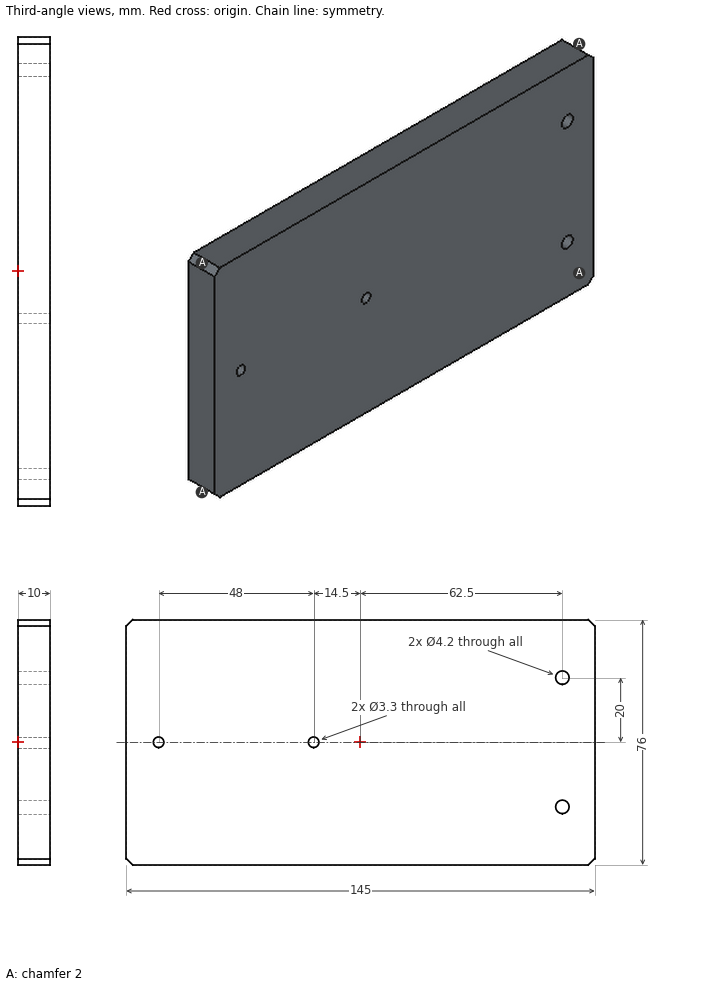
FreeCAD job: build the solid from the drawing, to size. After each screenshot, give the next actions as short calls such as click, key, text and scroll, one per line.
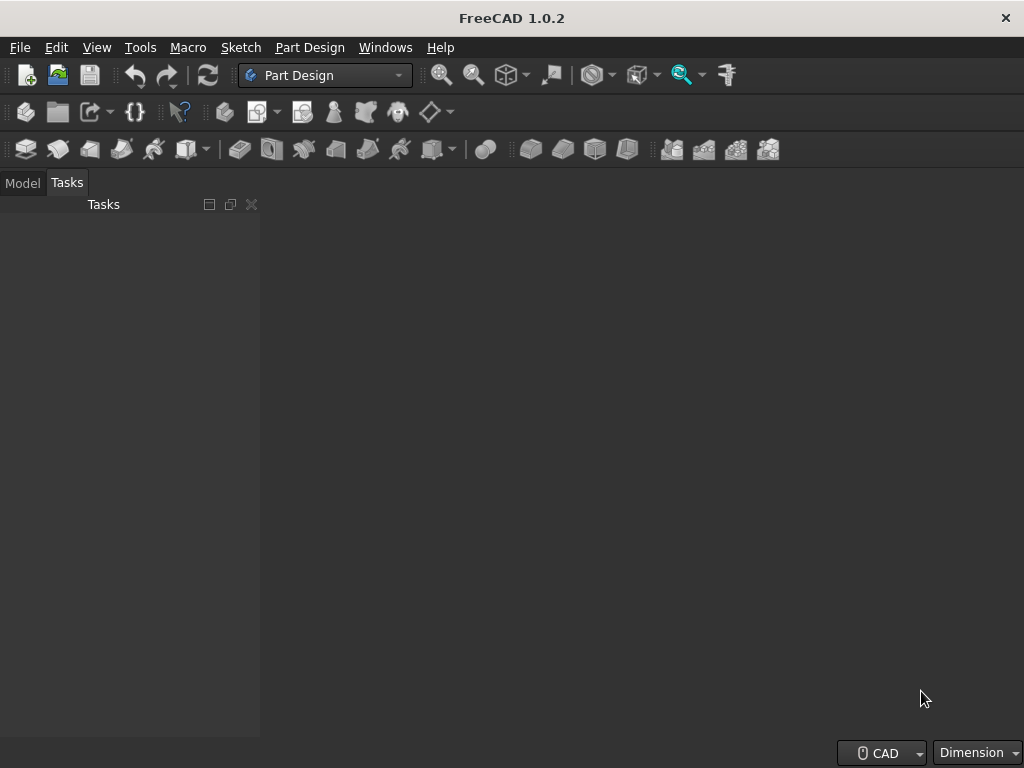
key(ctrl+n)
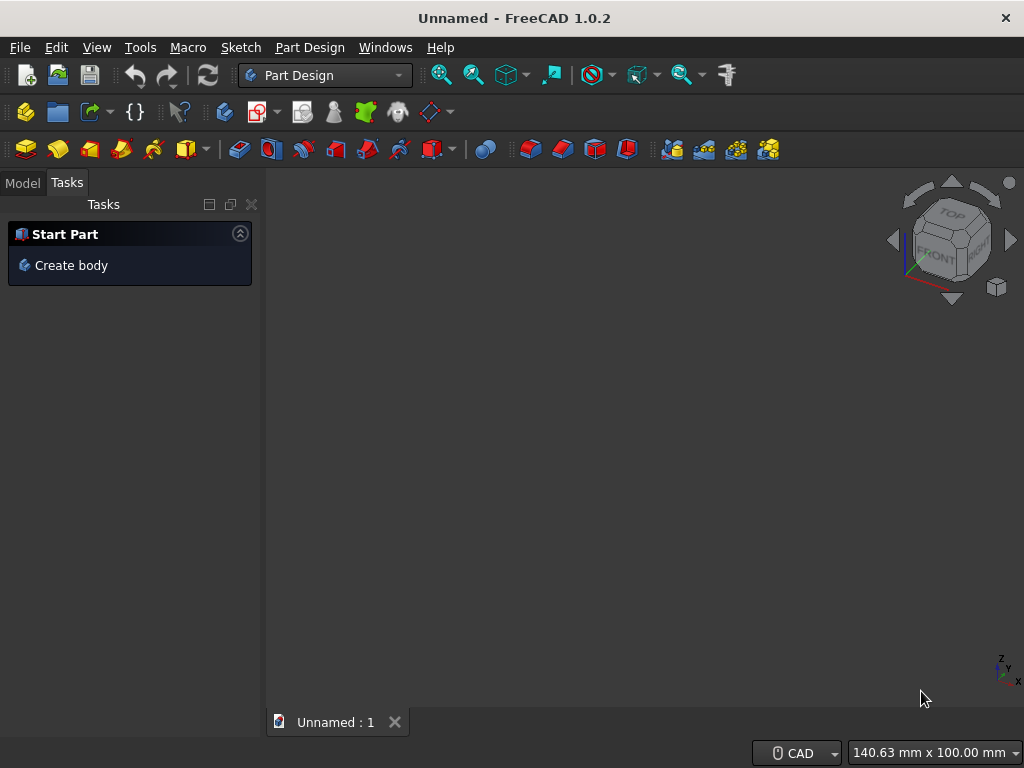
click(258, 112)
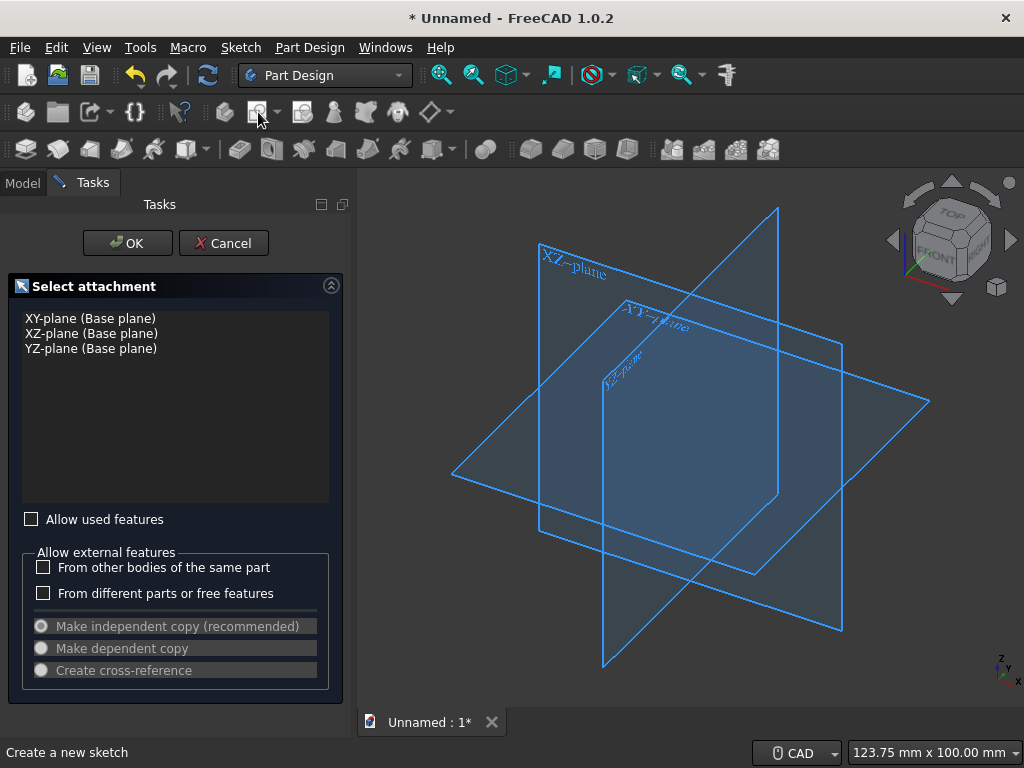
click(82, 348)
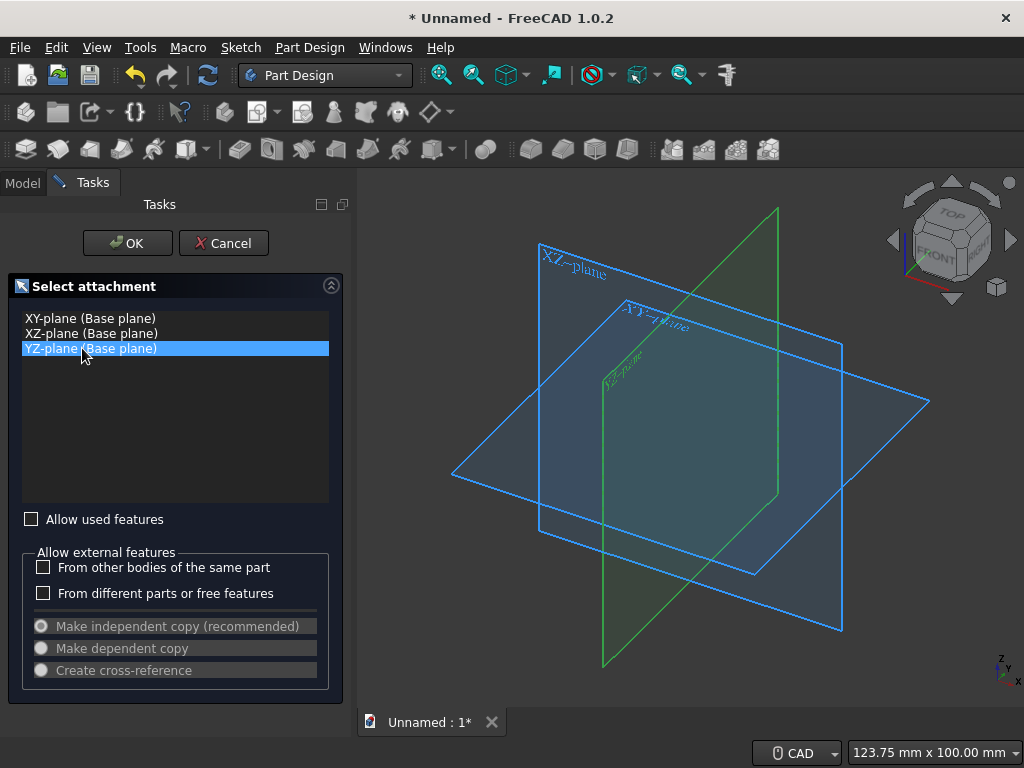
click(128, 243)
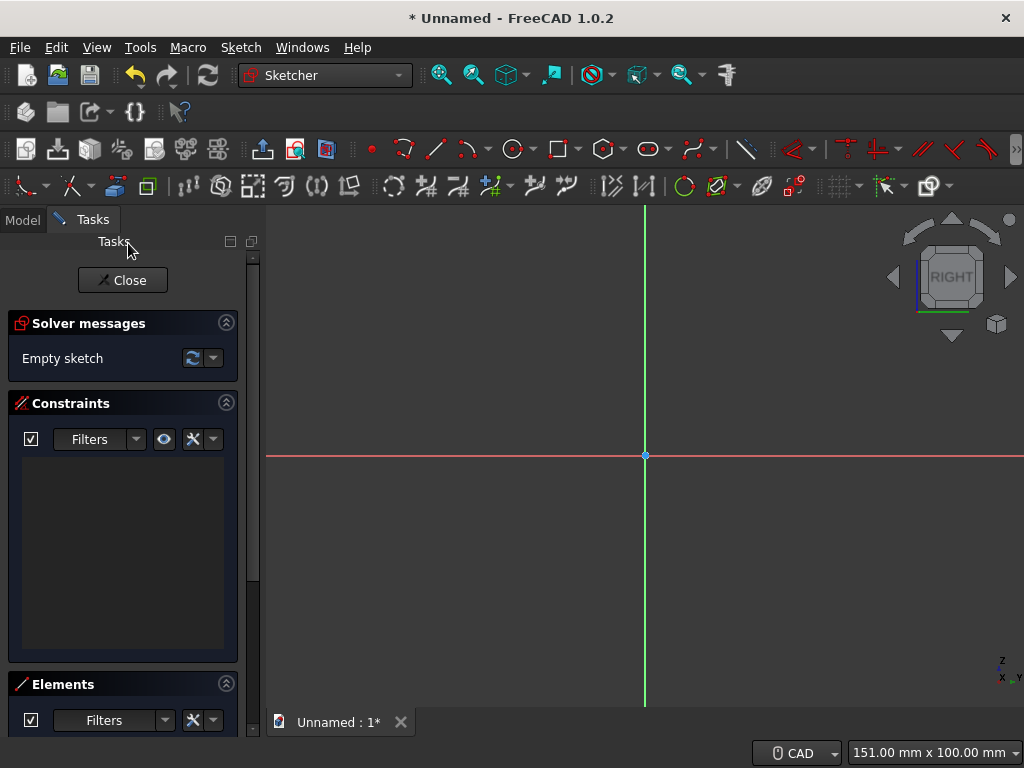
scroll(493, 456, down, 3)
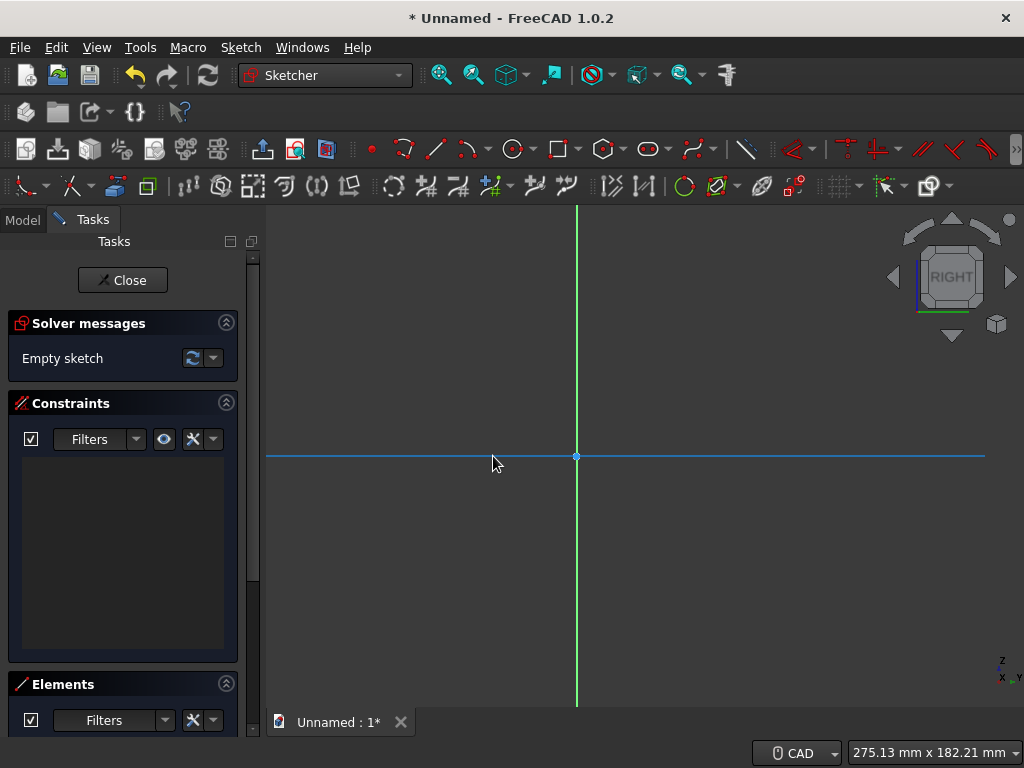
key(g)
key(v)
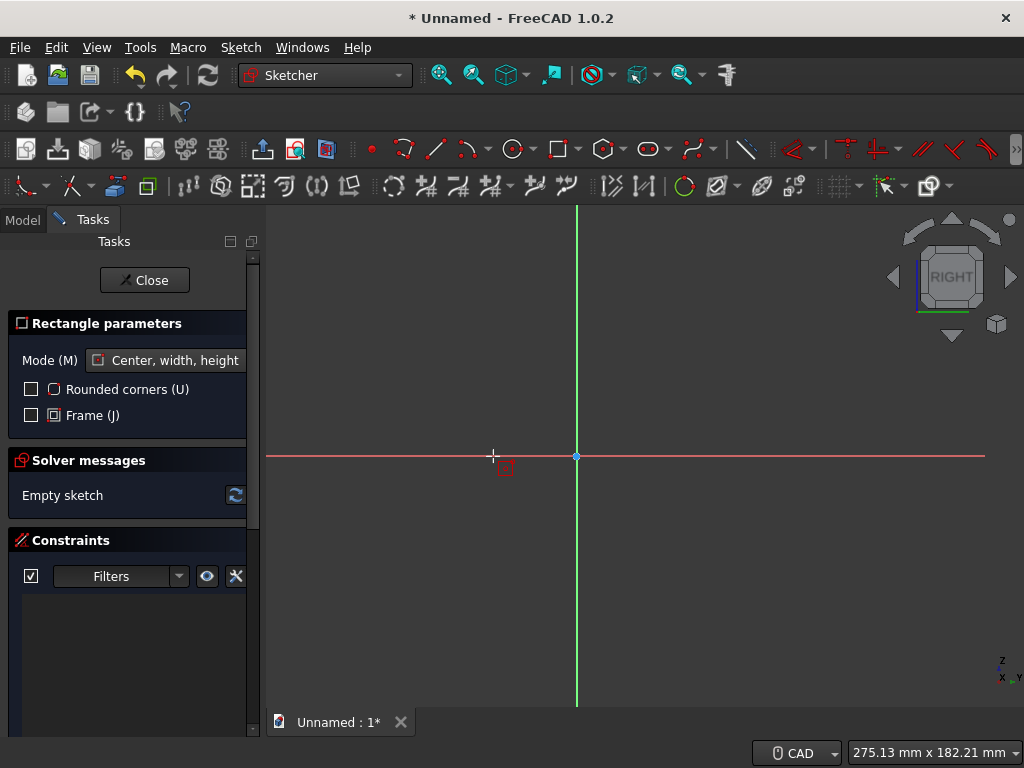
click(577, 456)
click(776, 352)
key(Escape)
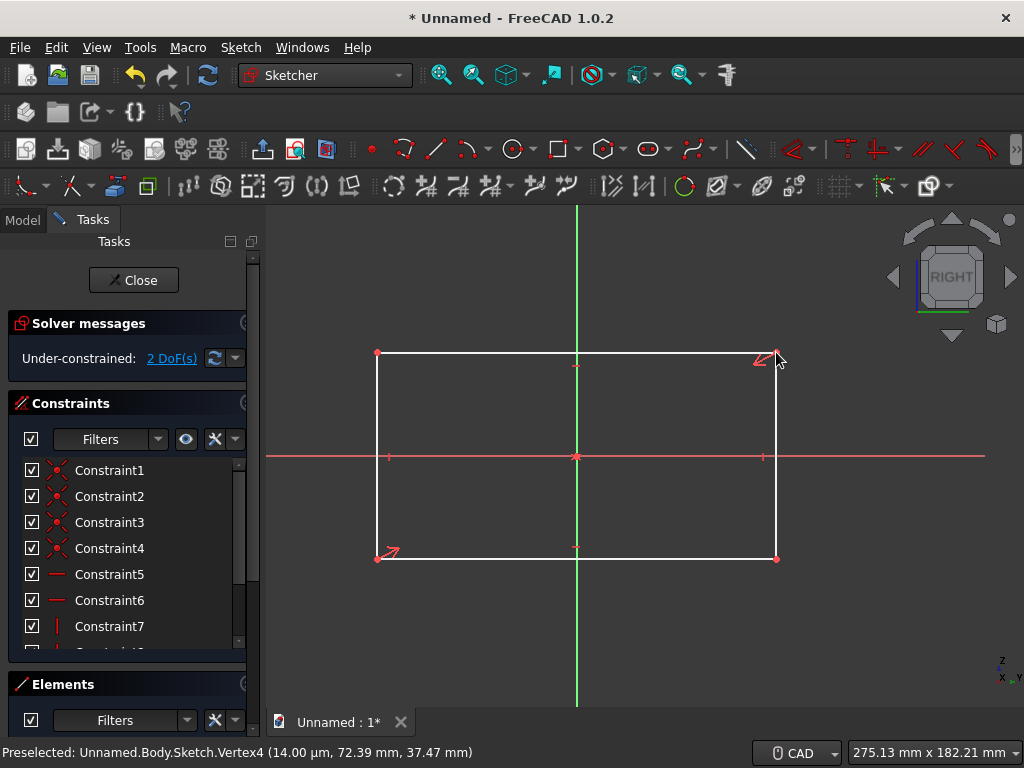
key(d)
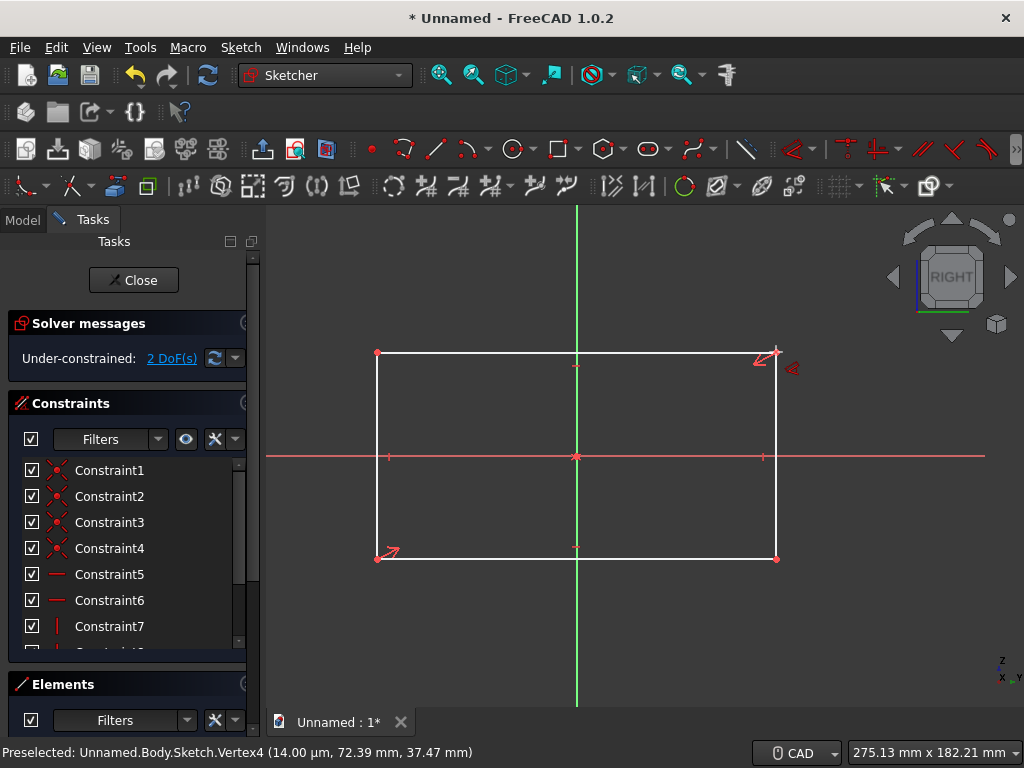
click(776, 498)
click(810, 409)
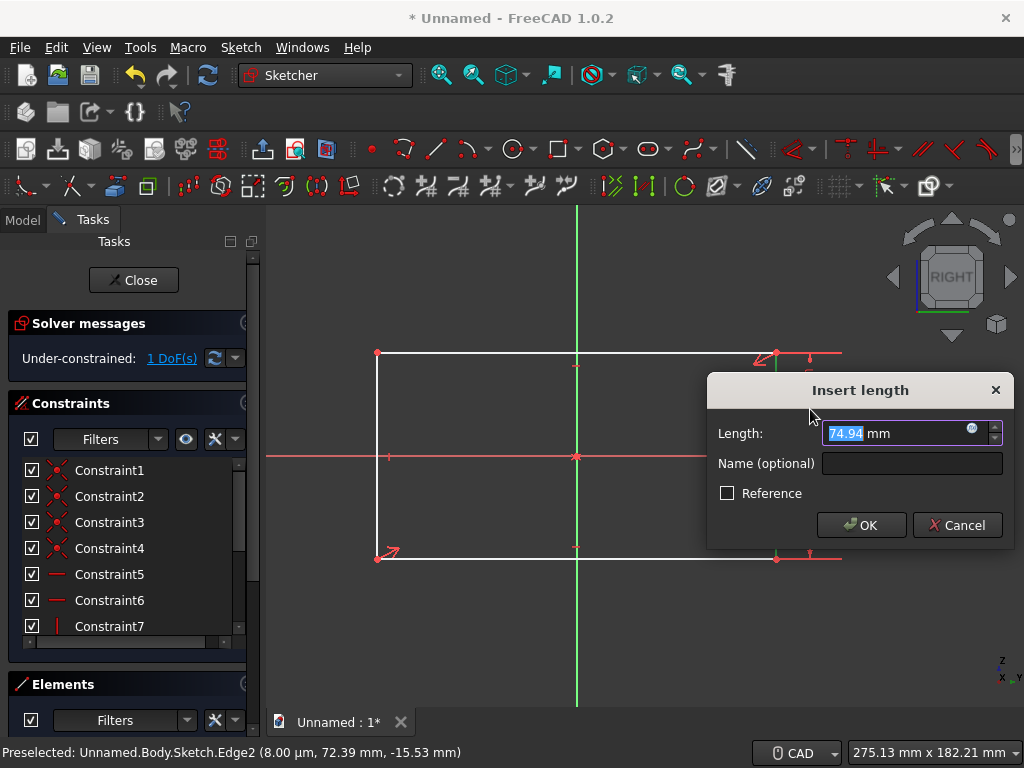
text(76)
key(Return)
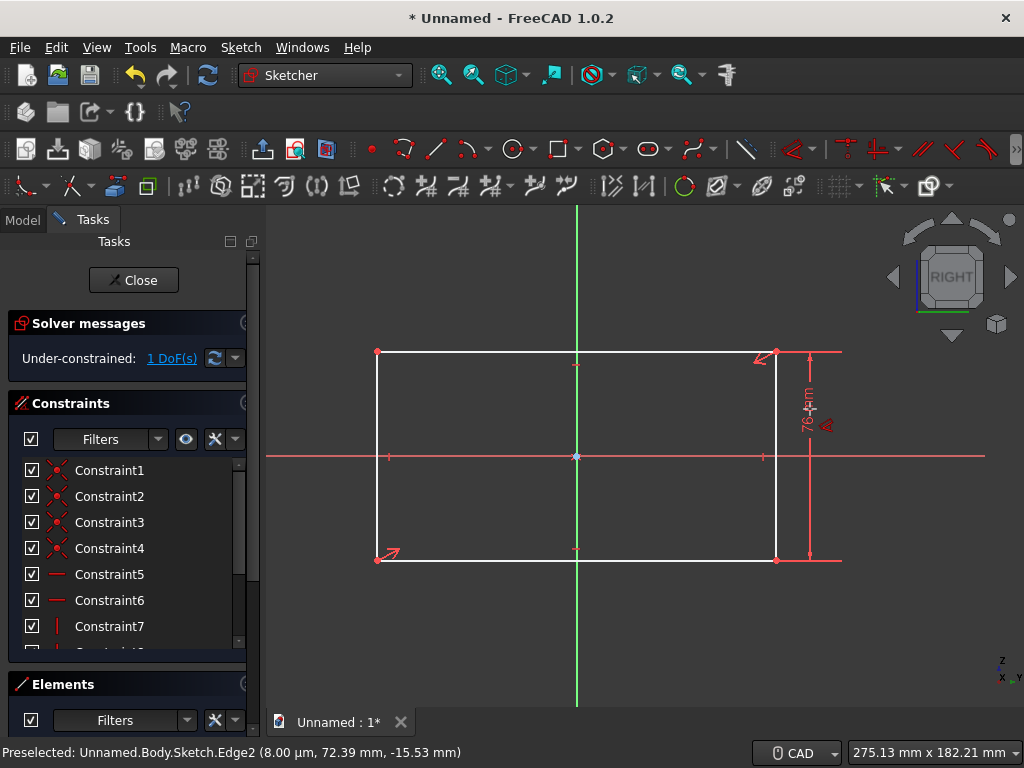
click(497, 561)
click(485, 595)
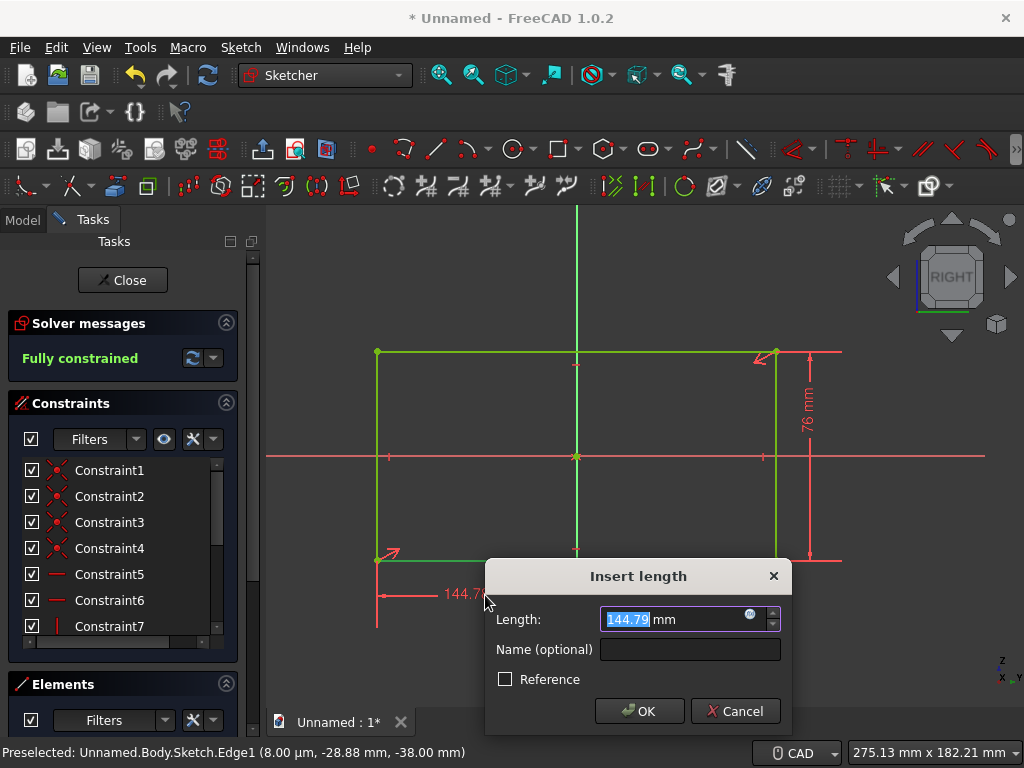
text(145)
key(Return)
key(Escape)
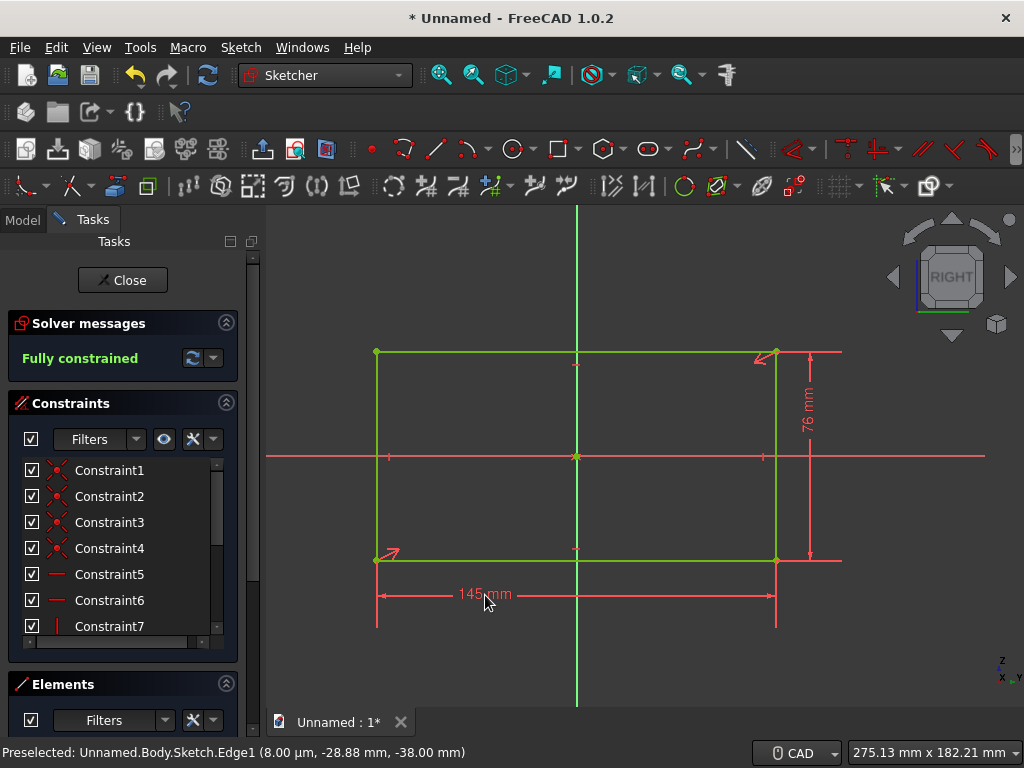
click(123, 280)